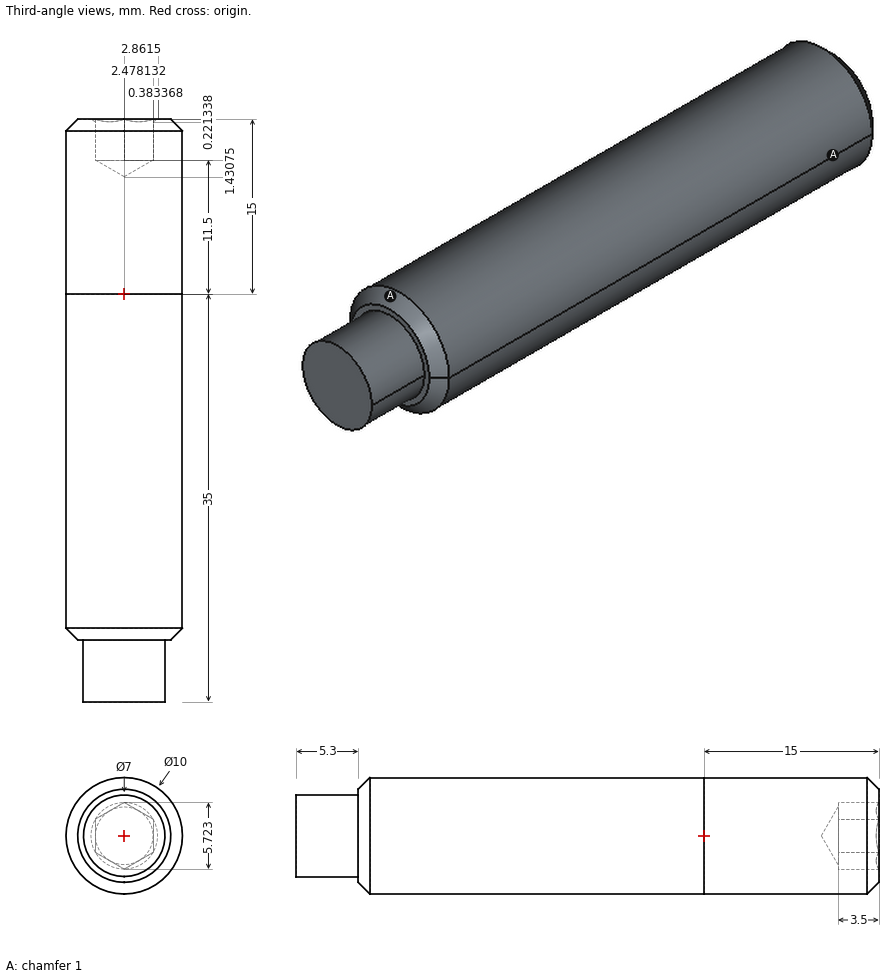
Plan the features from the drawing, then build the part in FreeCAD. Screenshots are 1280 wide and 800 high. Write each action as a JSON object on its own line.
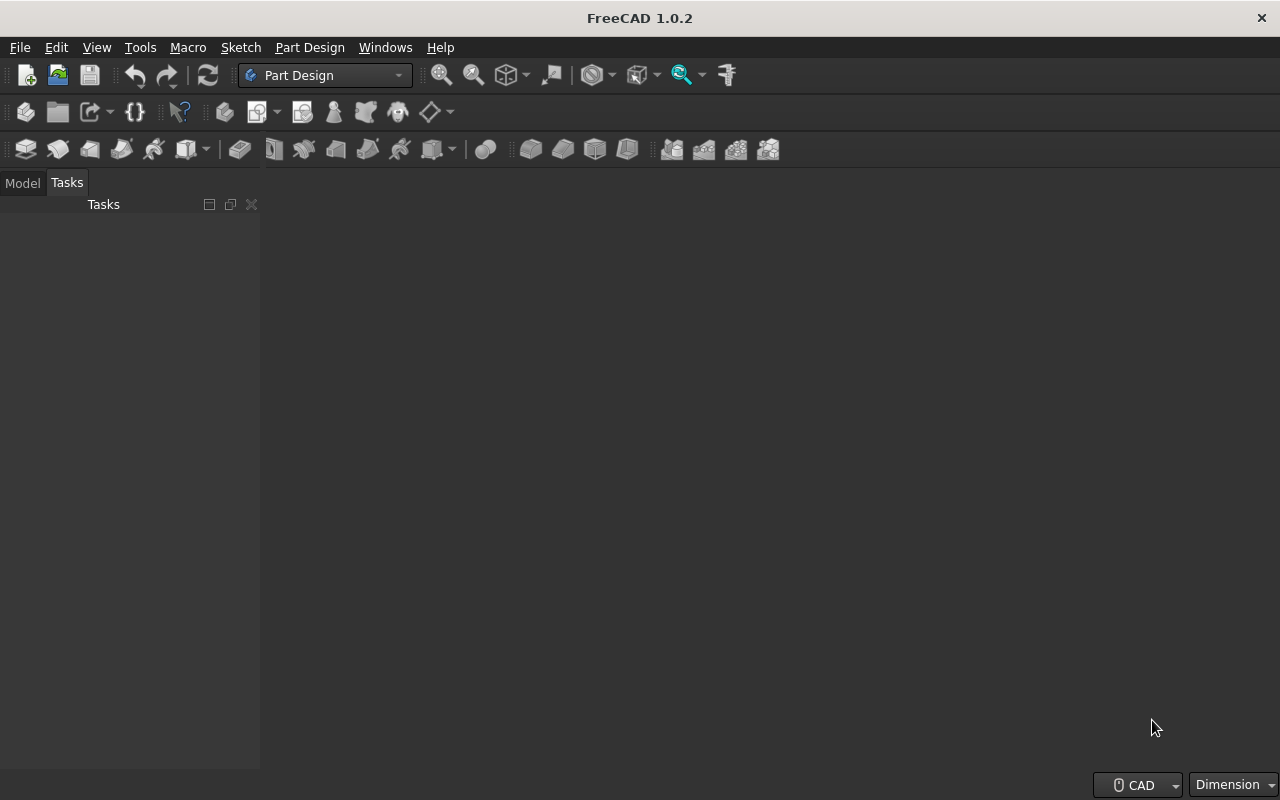
{"action": "left_click", "coordinate": [26, 76]}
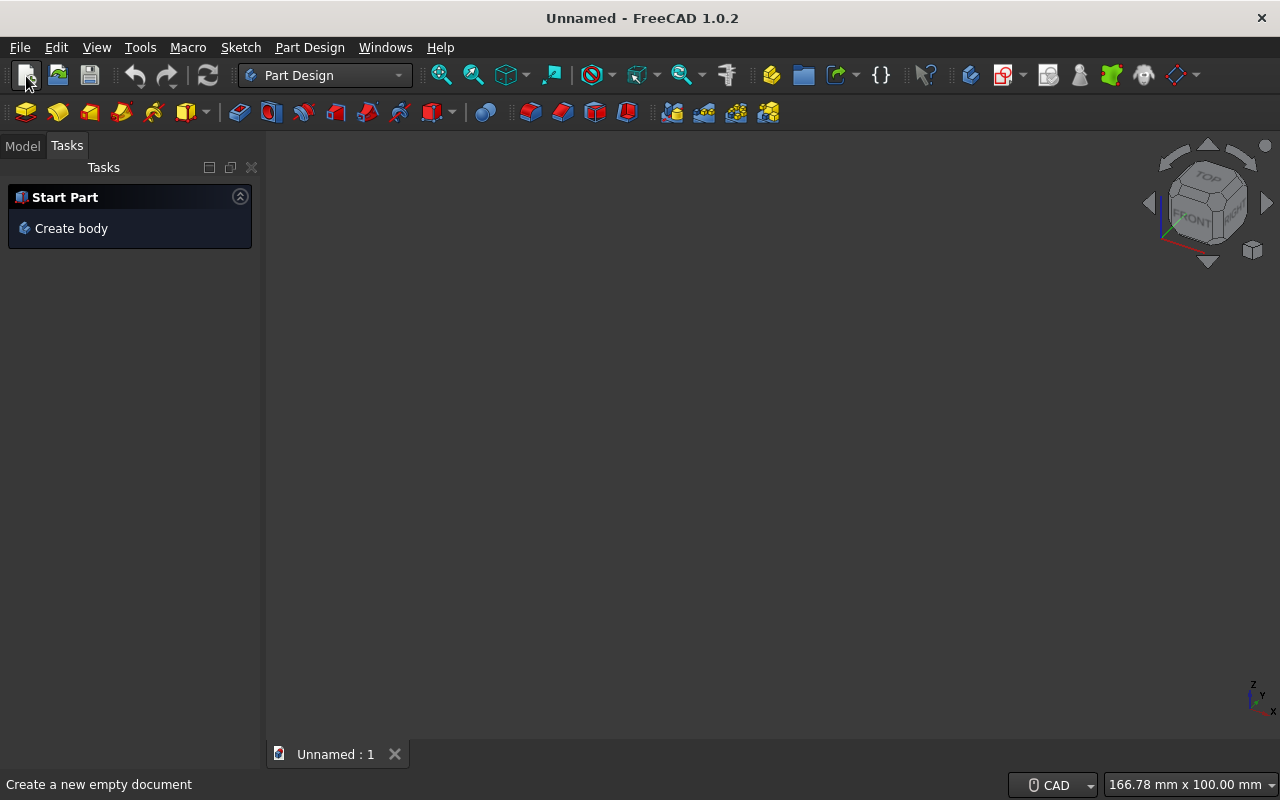
{"action": "left_click", "coordinate": [1004, 76]}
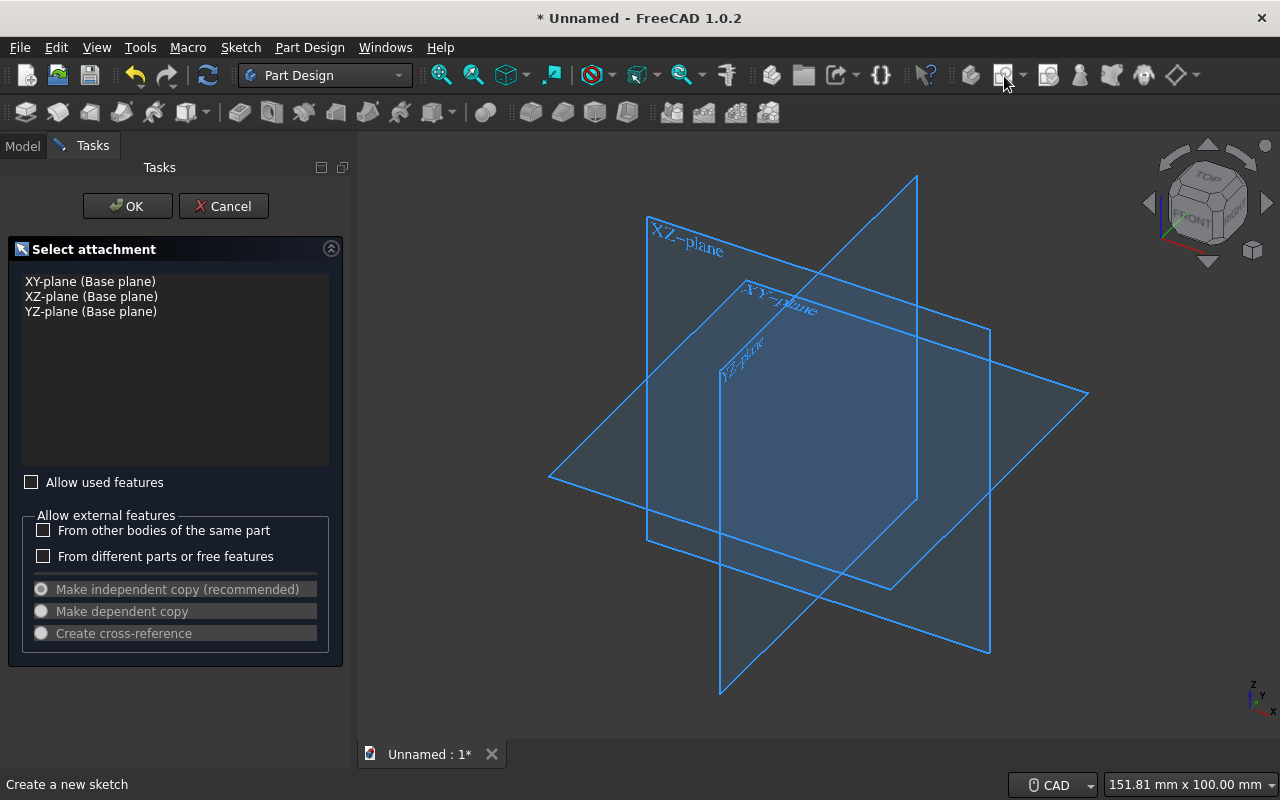
{"action": "left_click", "coordinate": [82, 296]}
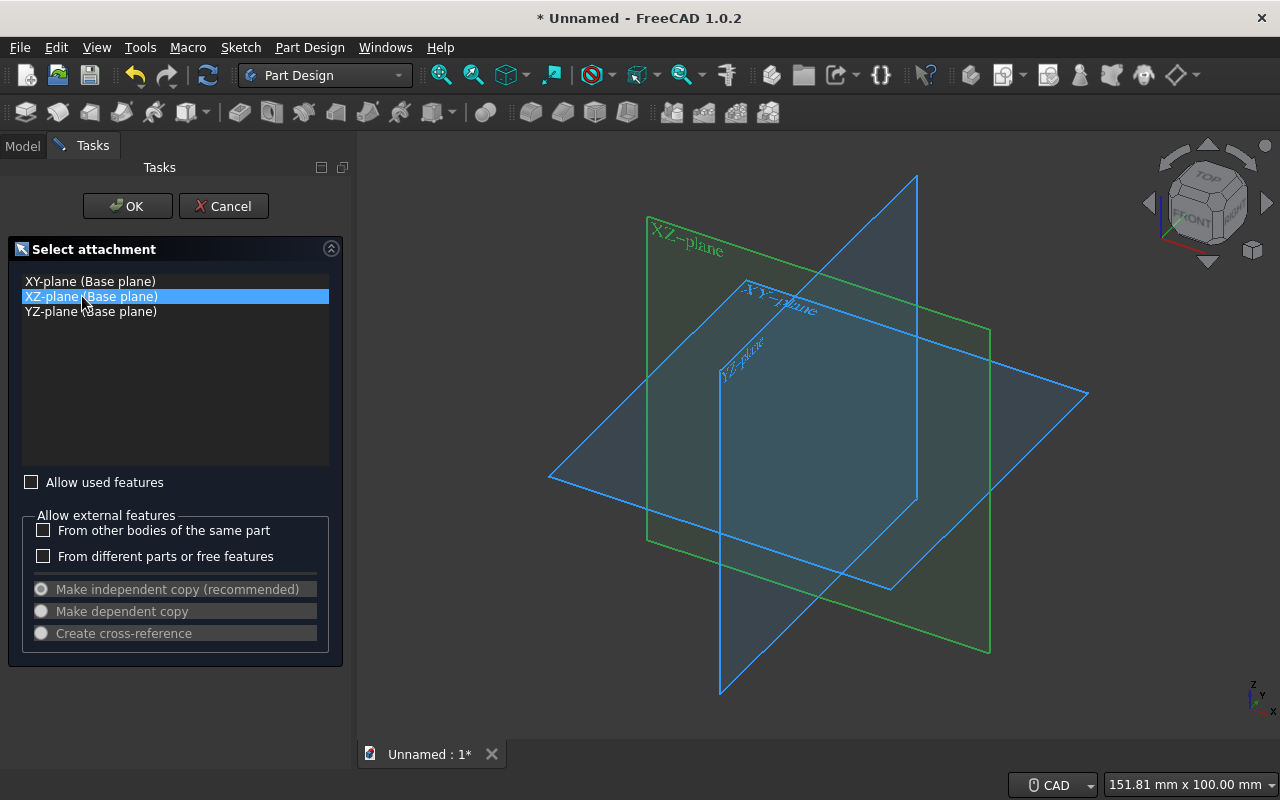
{"action": "left_click", "coordinate": [128, 206]}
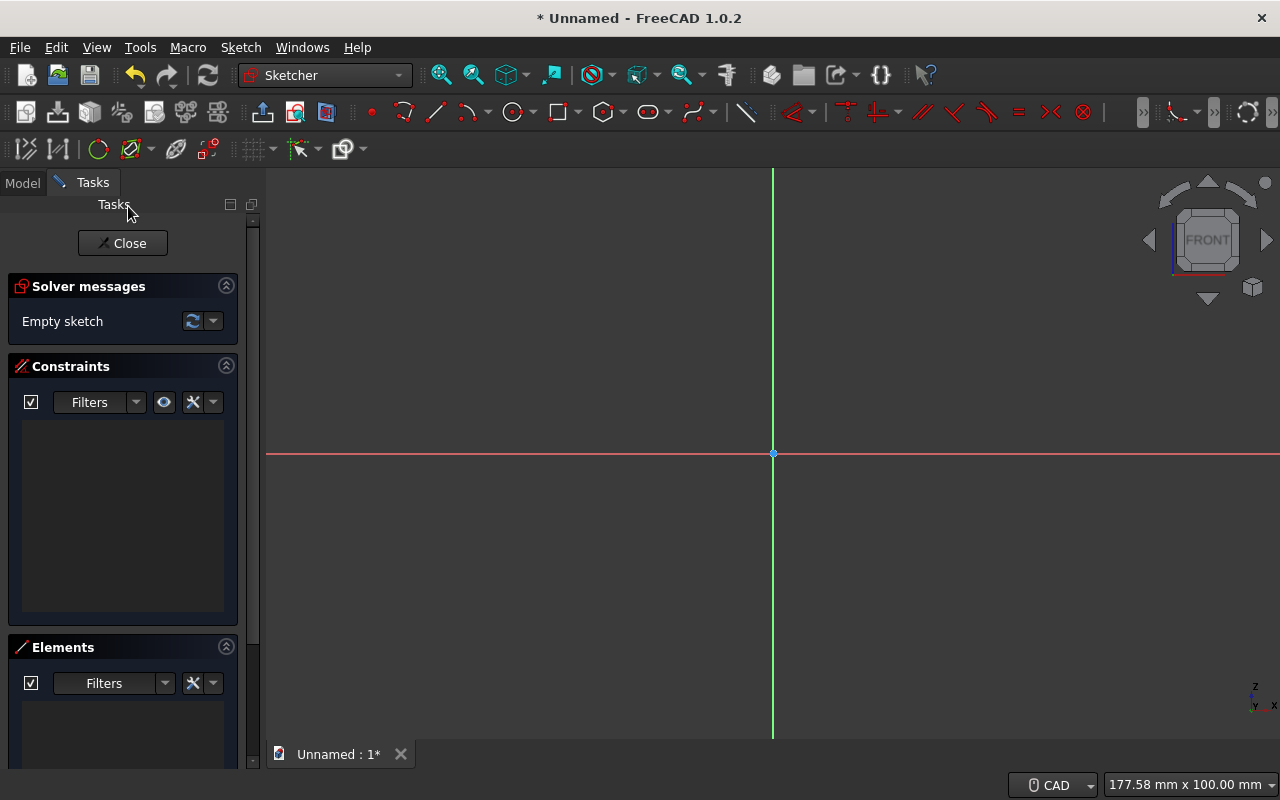
{"action": "scroll", "coordinate": [787, 454], "scroll_direction": "up", "scroll_amount": 9}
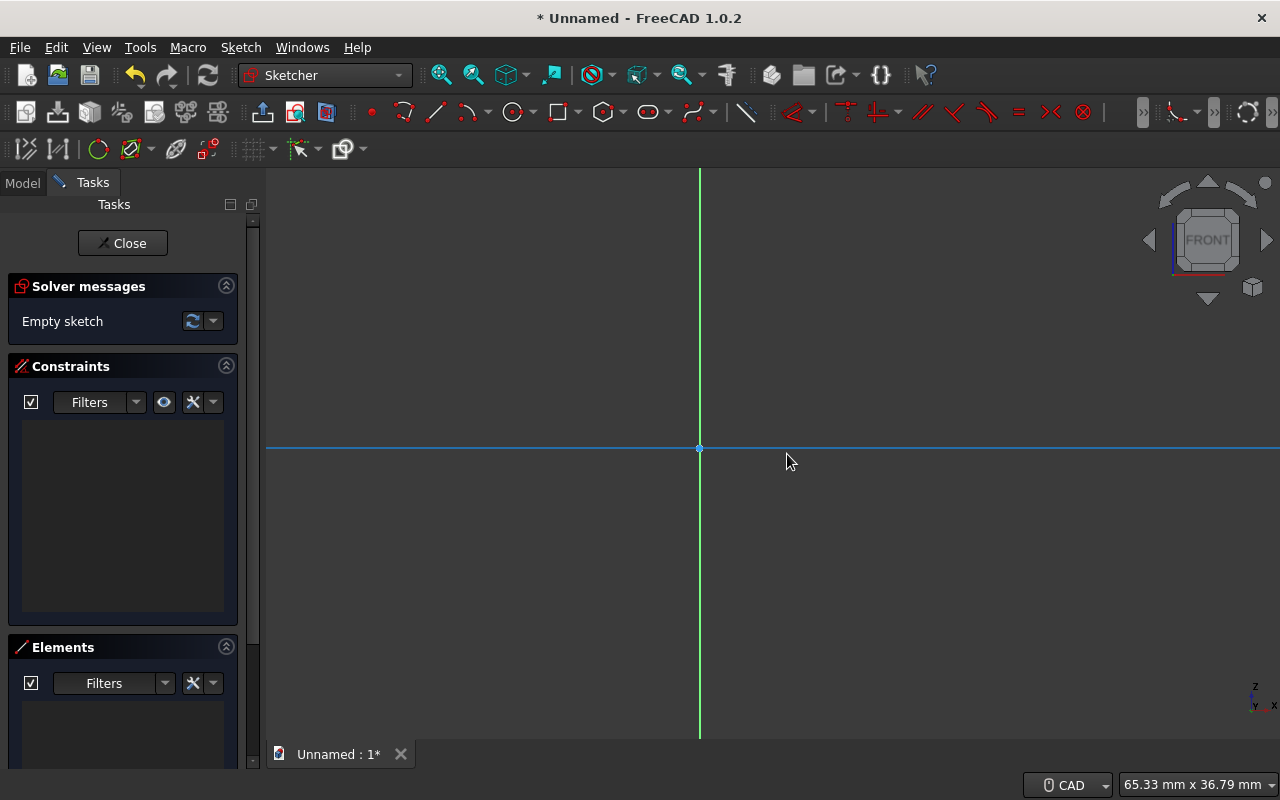
{"action": "left_click", "coordinate": [514, 112]}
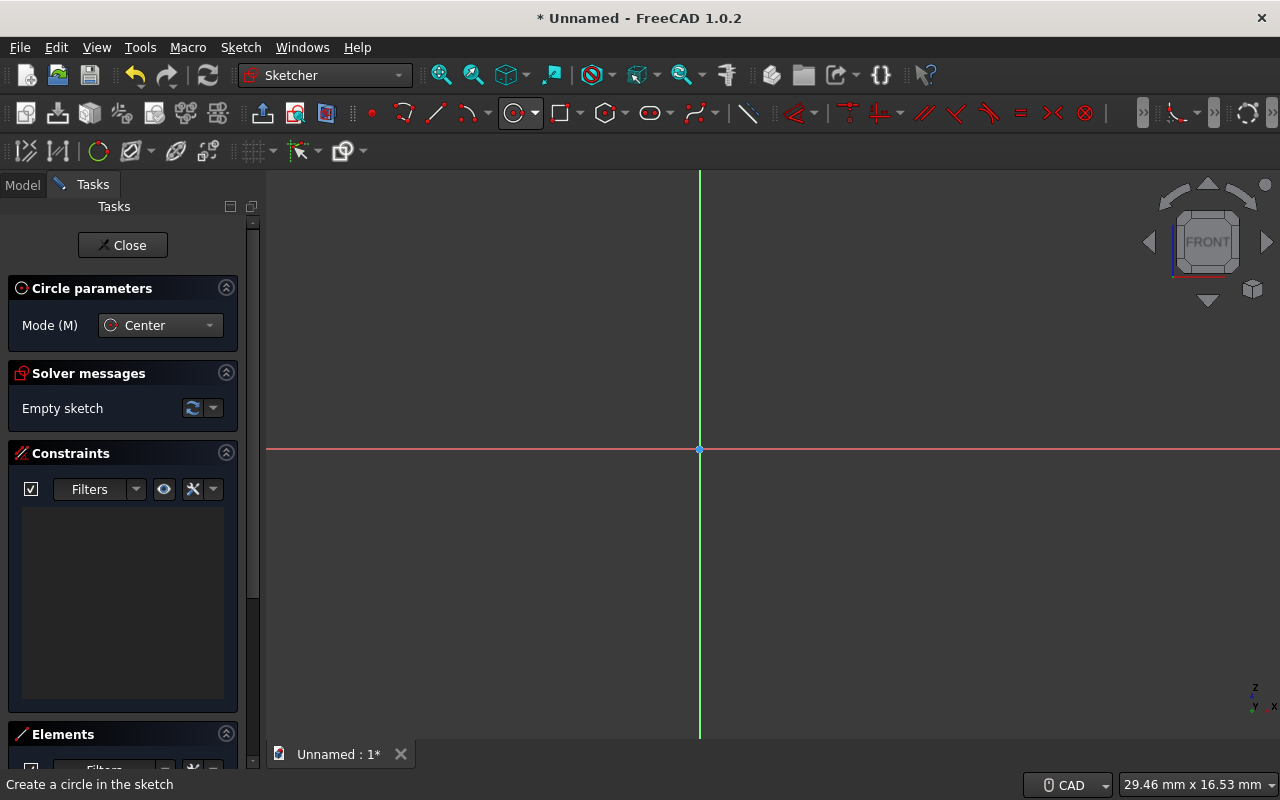
{"action": "left_click", "coordinate": [700, 449]}
{"action": "left_click", "coordinate": [822, 328]}
{"action": "key", "text": "Escape"}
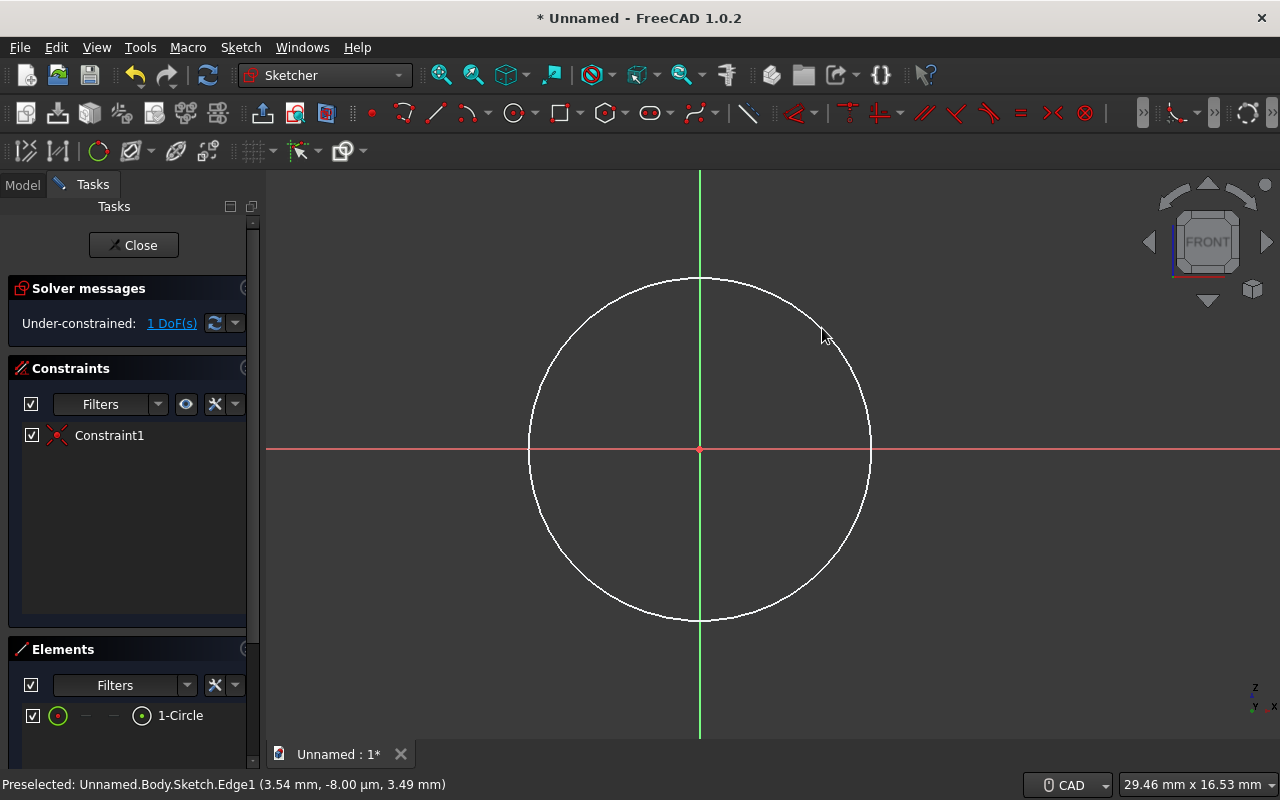
{"action": "left_click", "coordinate": [821, 328]}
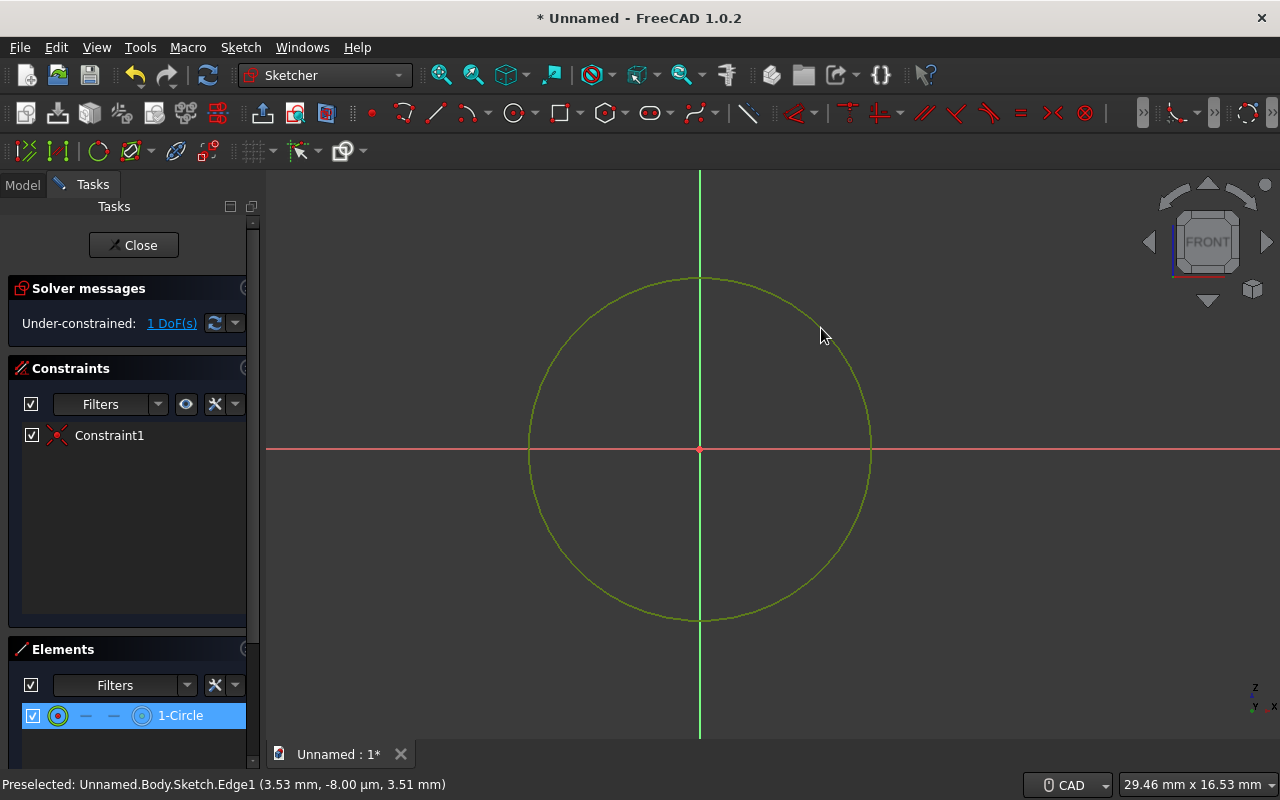
{"action": "key", "text": "k o"}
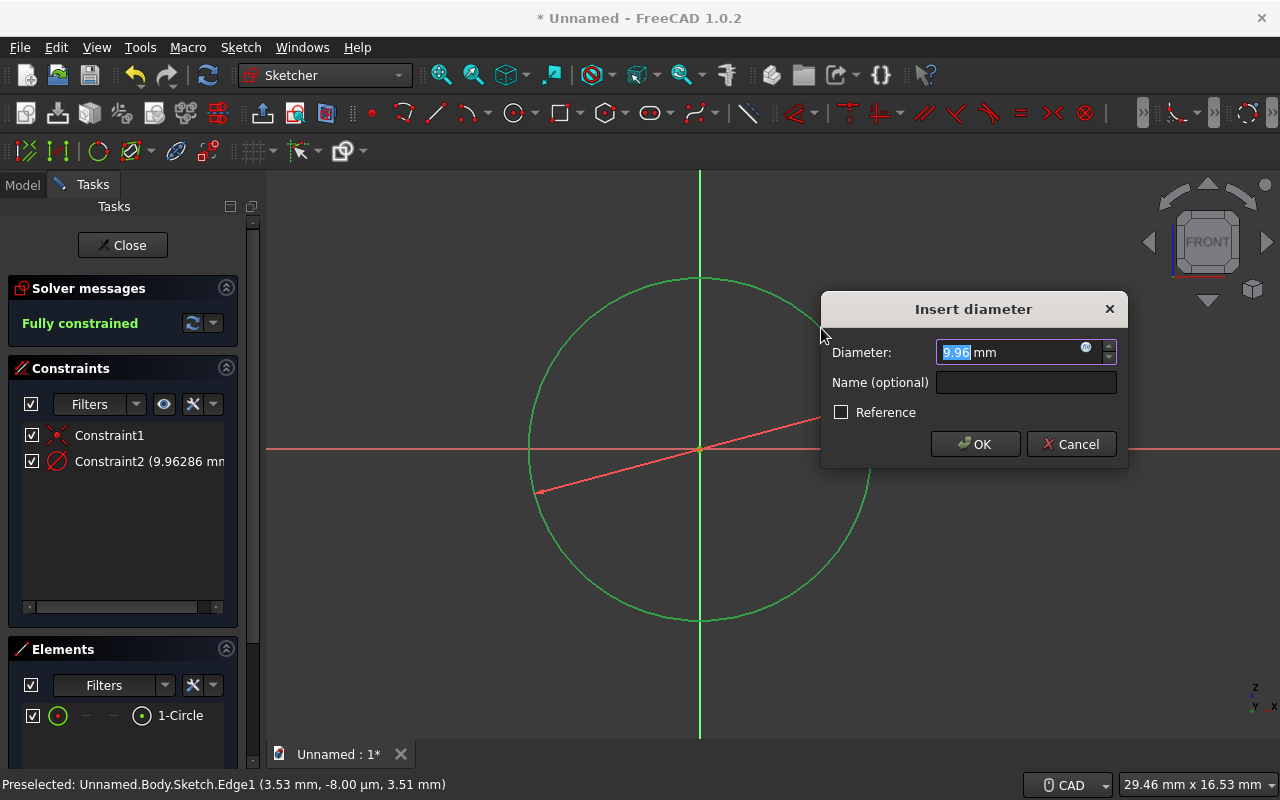
{"action": "type", "text": "10"}
{"action": "key", "text": "Return"}